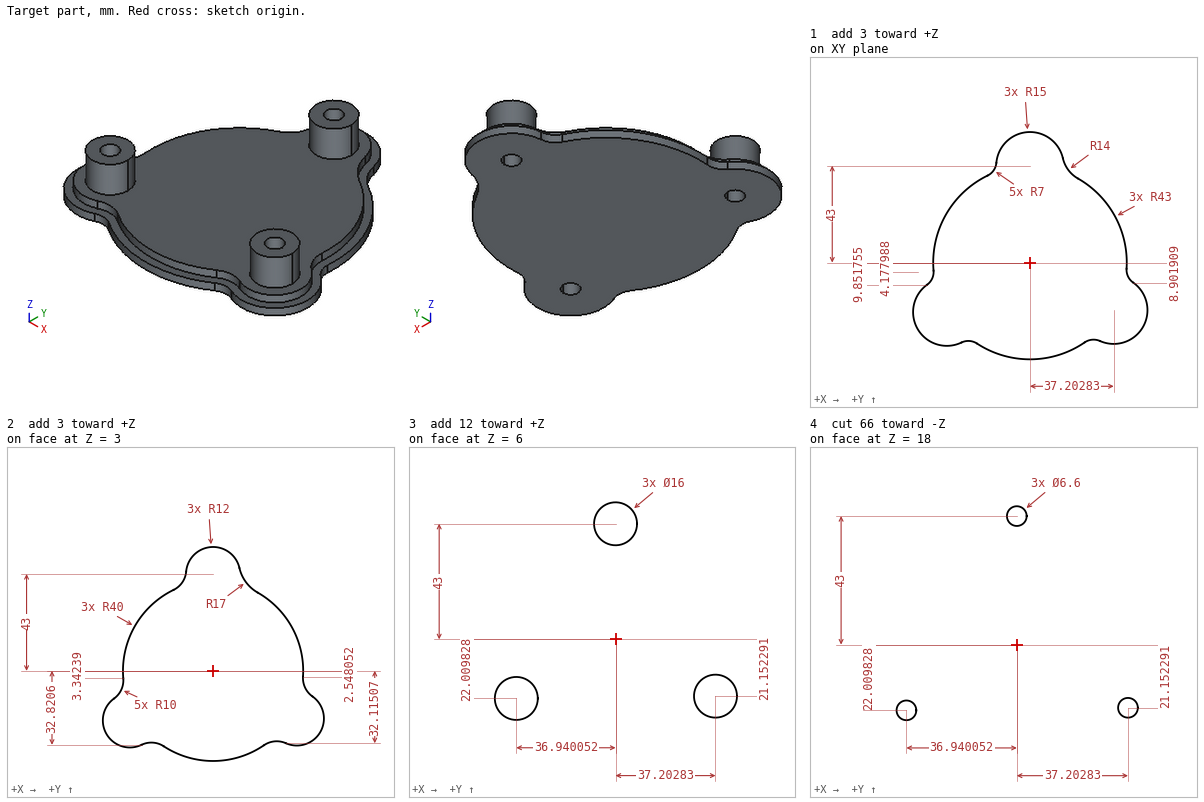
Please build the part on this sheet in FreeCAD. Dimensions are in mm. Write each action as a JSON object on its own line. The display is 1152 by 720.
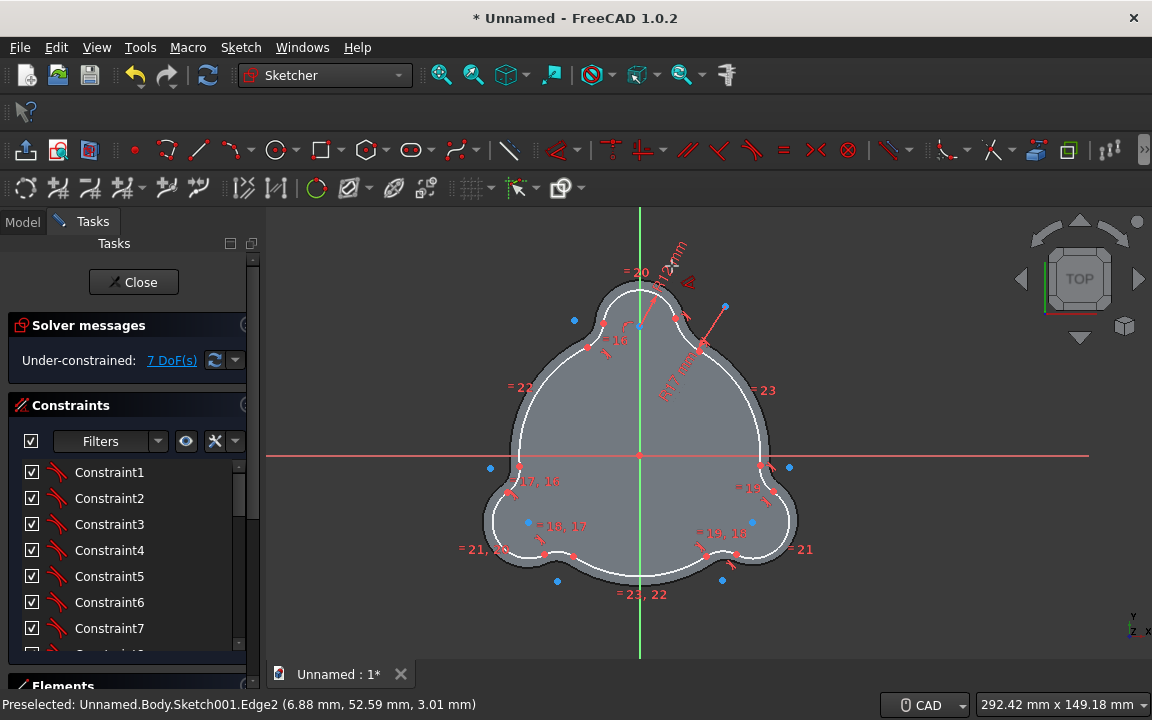
{"action": "scroll", "coordinate": [595, 342], "scroll_direction": "up", "scroll_amount": 3}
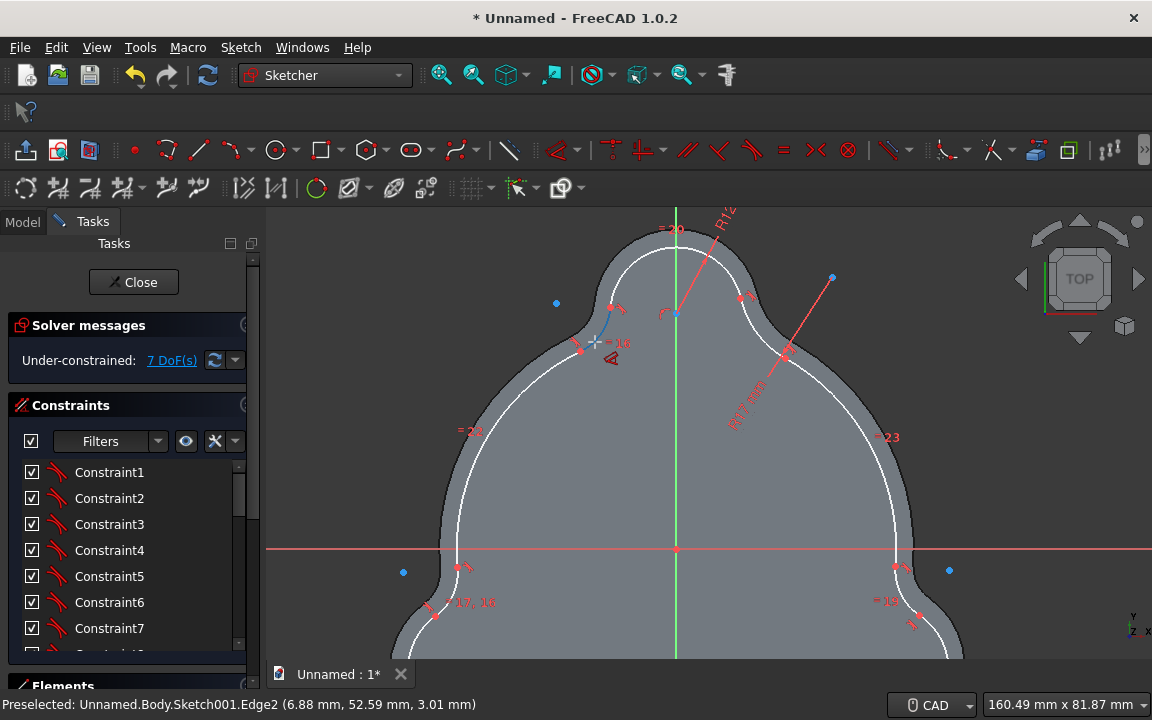
{"action": "left_click", "coordinate": [594, 342]}
{"action": "left_click", "coordinate": [616, 365]}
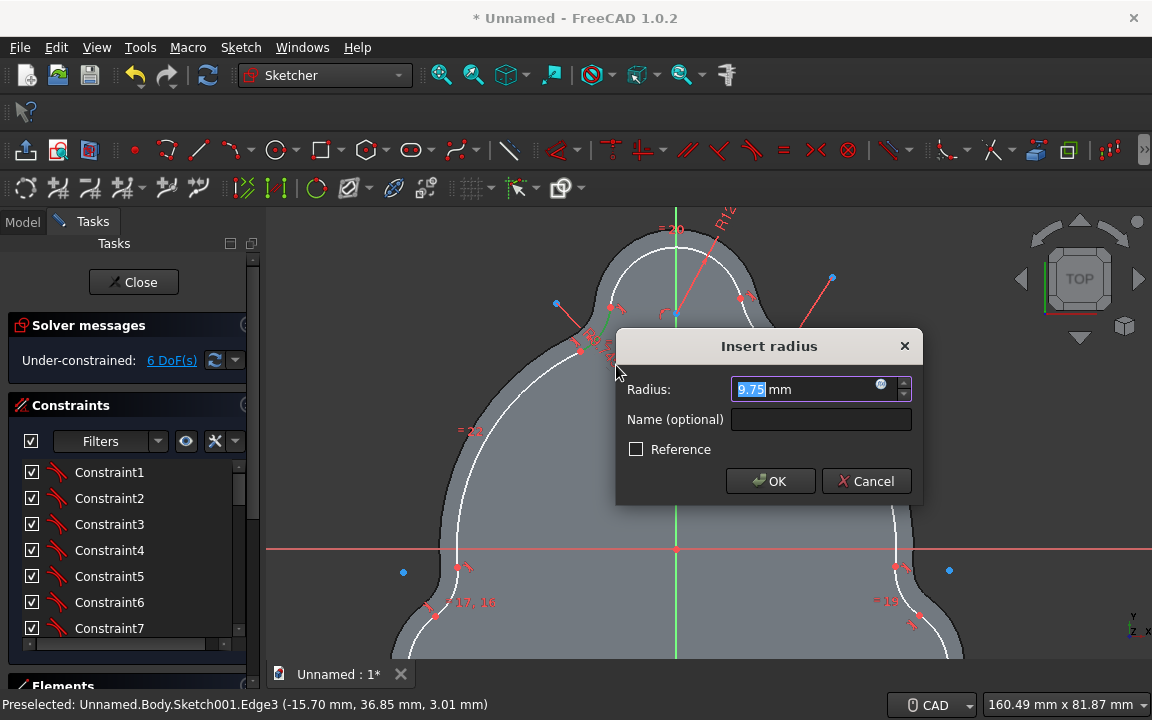
{"action": "type", "text": "10"}
{"action": "key", "text": "Return"}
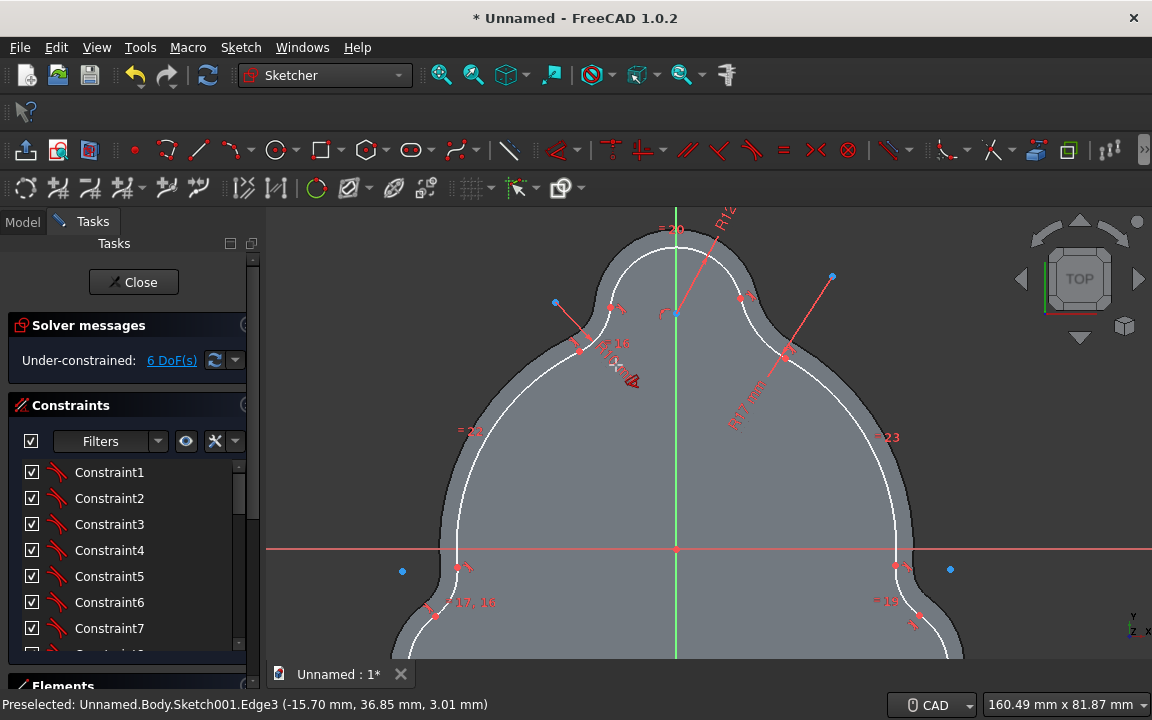
{"action": "left_click", "coordinate": [517, 398]}
{"action": "left_click", "coordinate": [494, 376]}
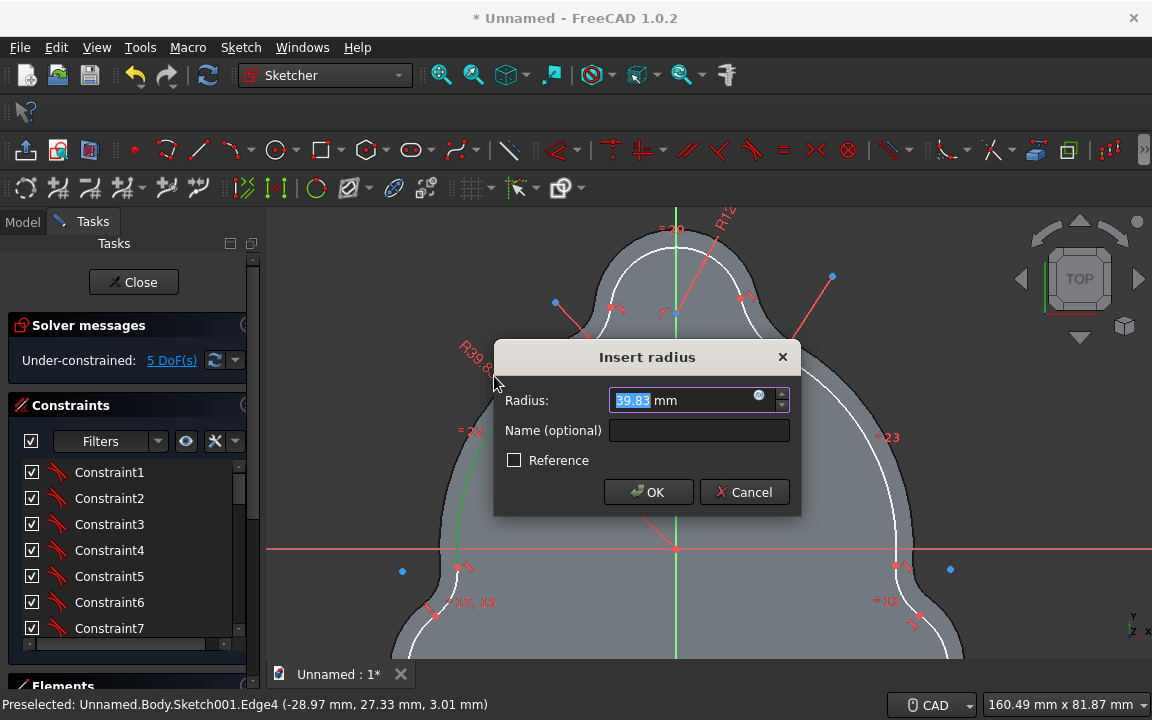
{"action": "type", "text": "40"}
{"action": "key", "text": "Return"}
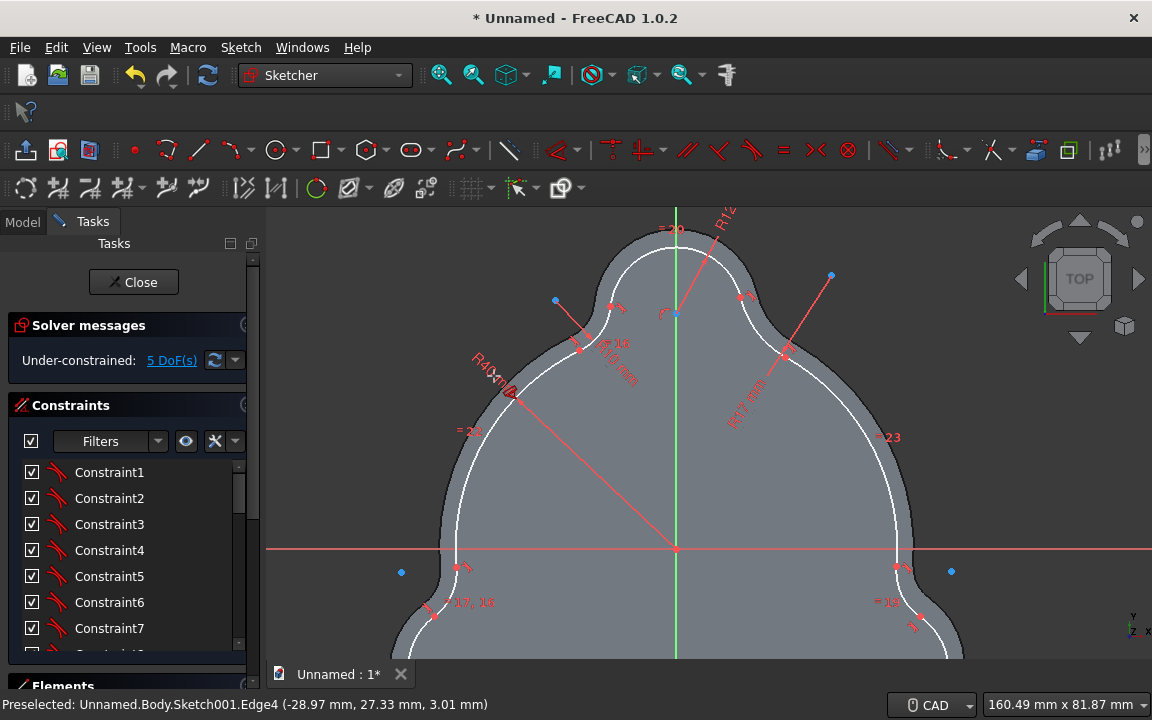
{"action": "left_click", "coordinate": [676, 314]}
{"action": "left_click", "coordinate": [642, 431]}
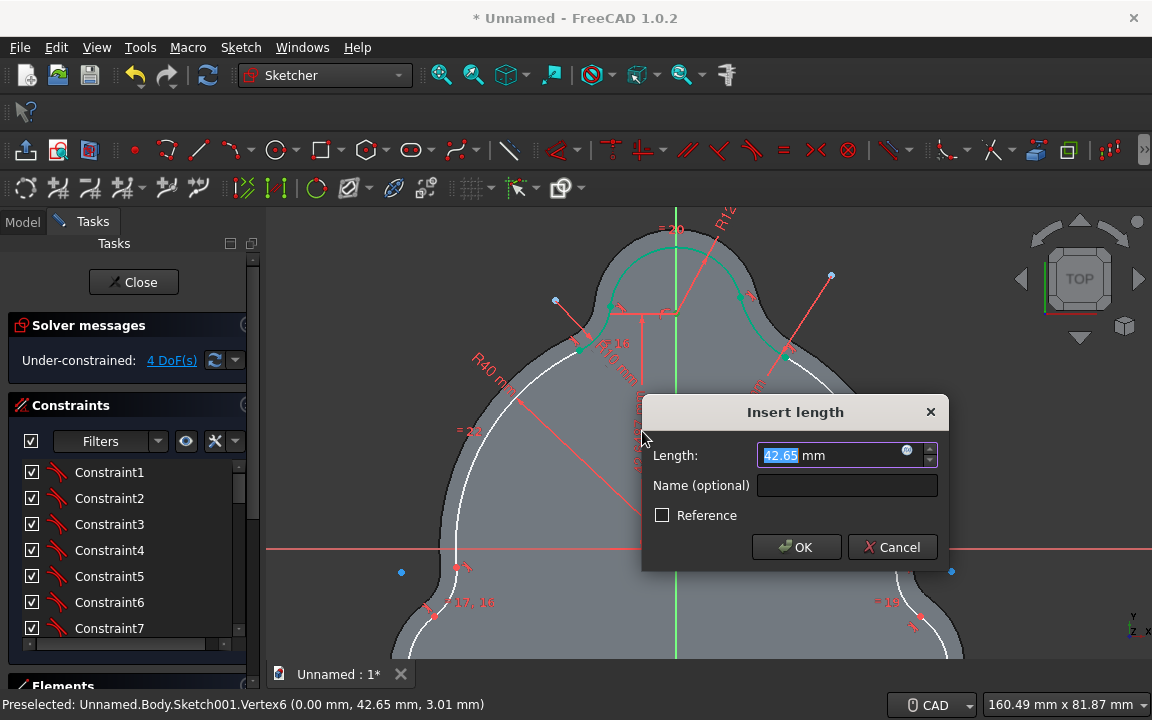
{"action": "type", "text": "43"}
{"action": "key", "text": "Return"}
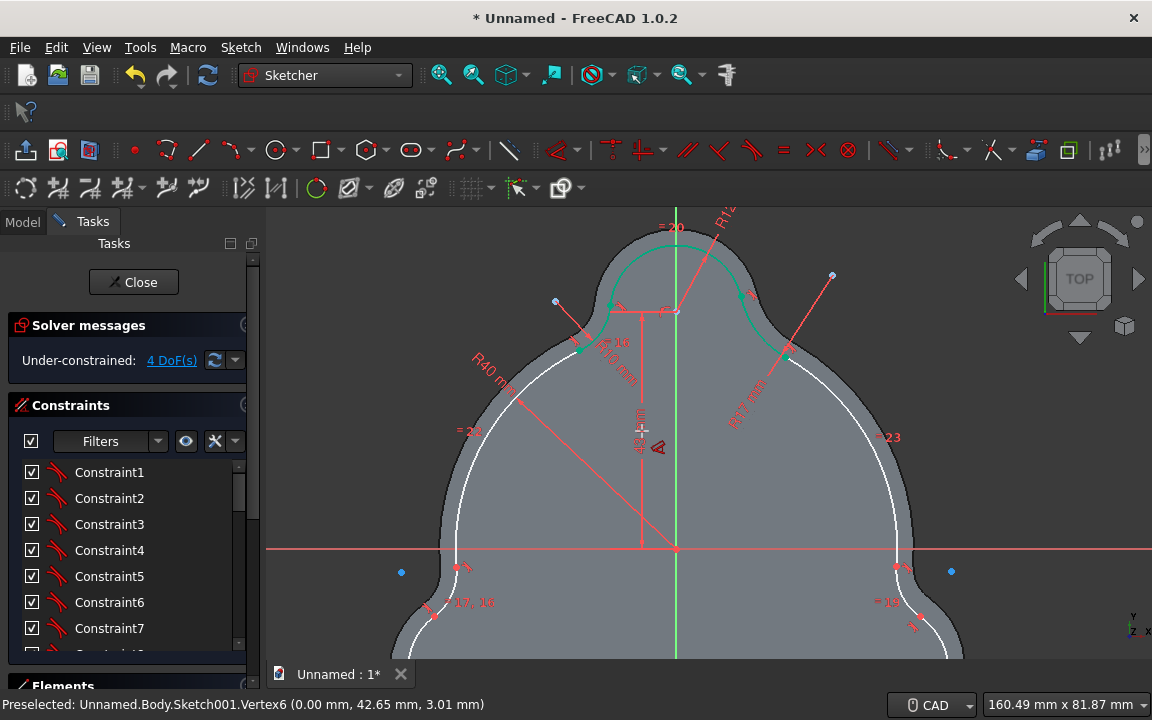
{"action": "scroll", "coordinate": [456, 568], "scroll_direction": "up", "scroll_amount": 4}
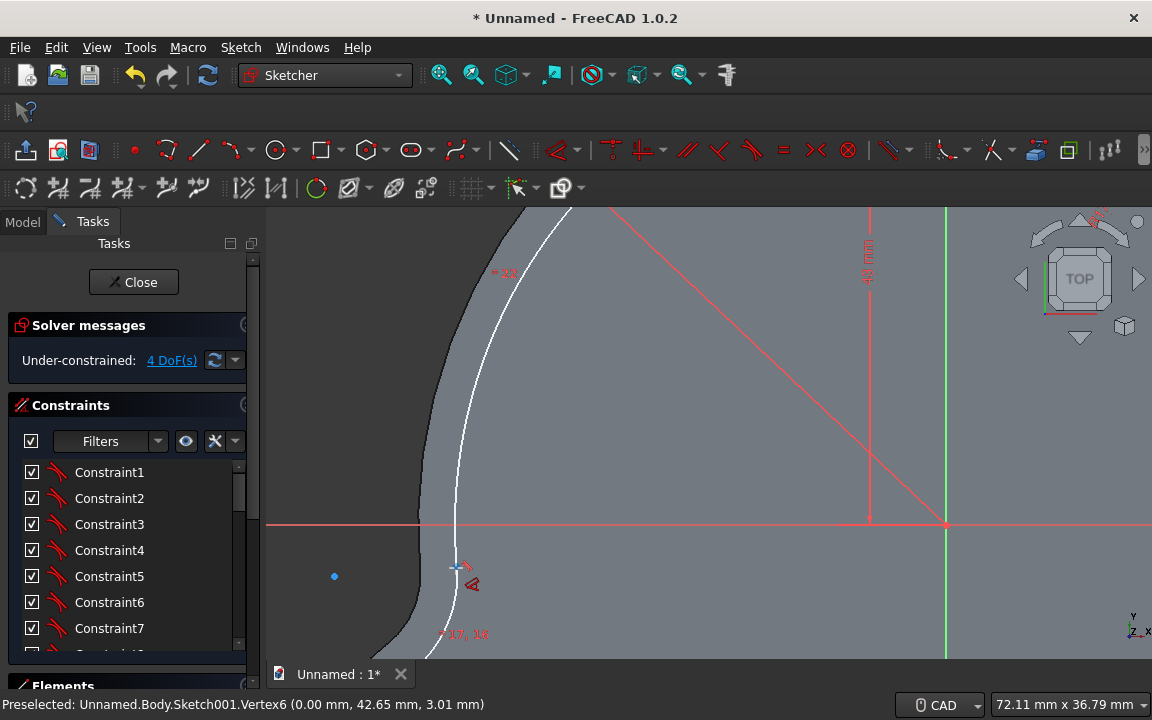
{"action": "left_click", "coordinate": [457, 566]}
{"action": "left_click", "coordinate": [423, 546]}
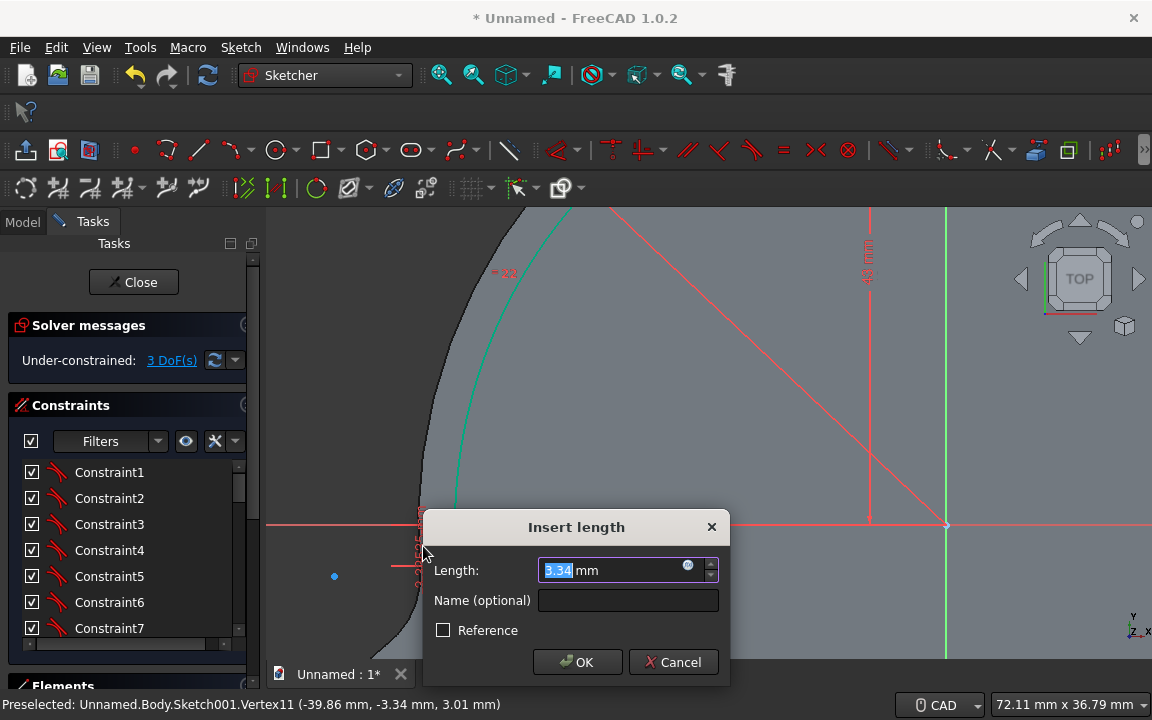
{"action": "type", "text": "3.34239"}
{"action": "key", "text": "Return"}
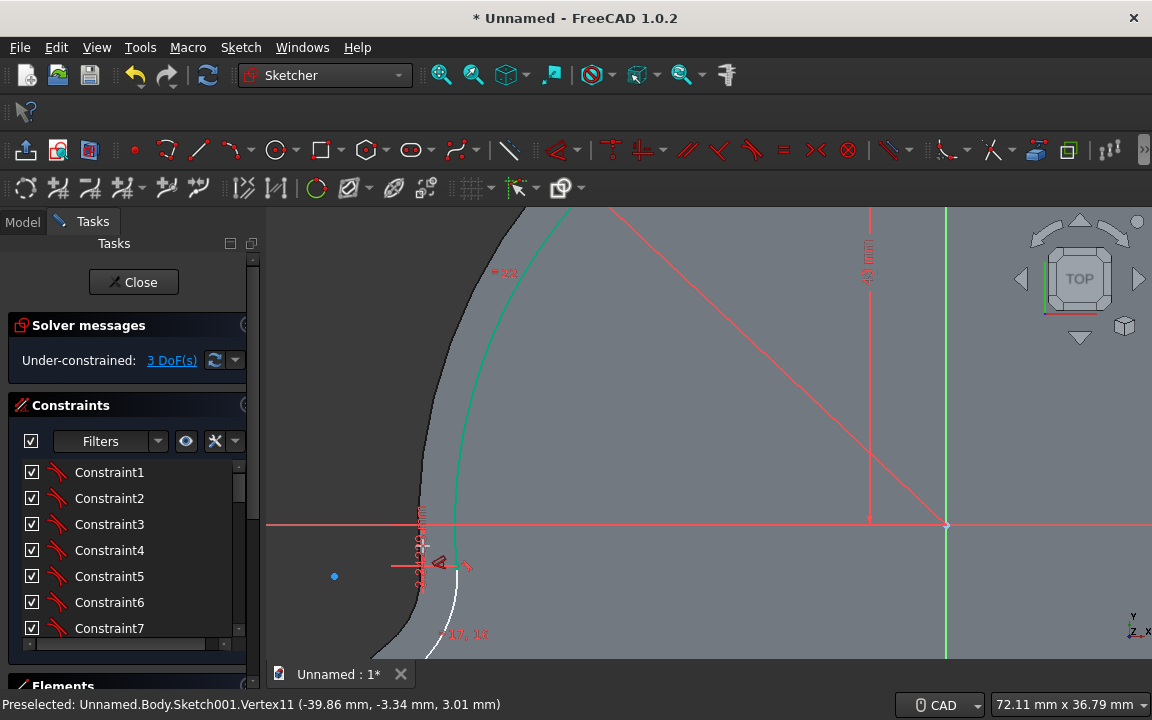
{"action": "scroll", "coordinate": [540, 433], "scroll_direction": "down", "scroll_amount": 7}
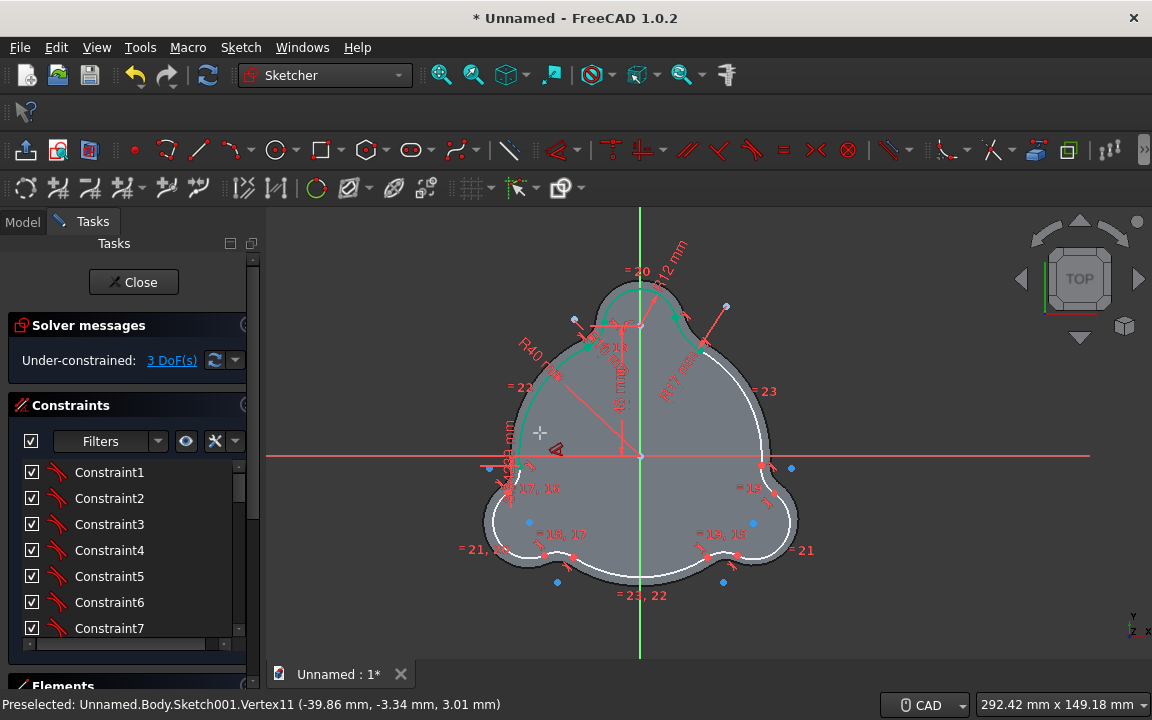
{"action": "left_click", "coordinate": [545, 555]}
{"action": "left_click", "coordinate": [511, 528]}